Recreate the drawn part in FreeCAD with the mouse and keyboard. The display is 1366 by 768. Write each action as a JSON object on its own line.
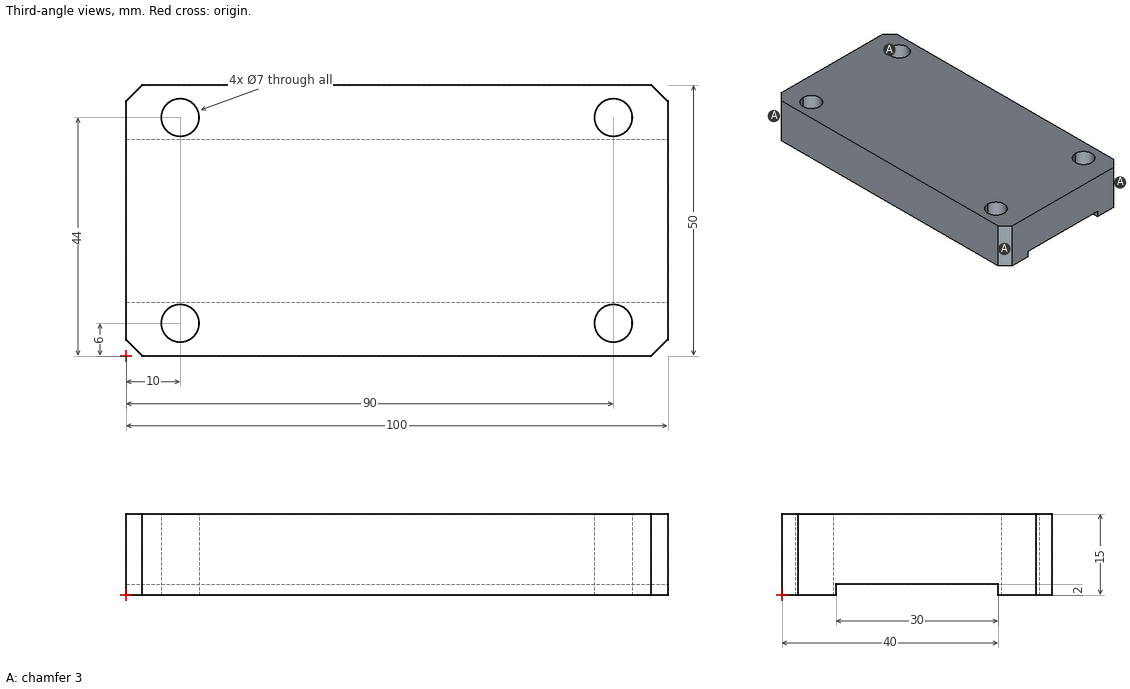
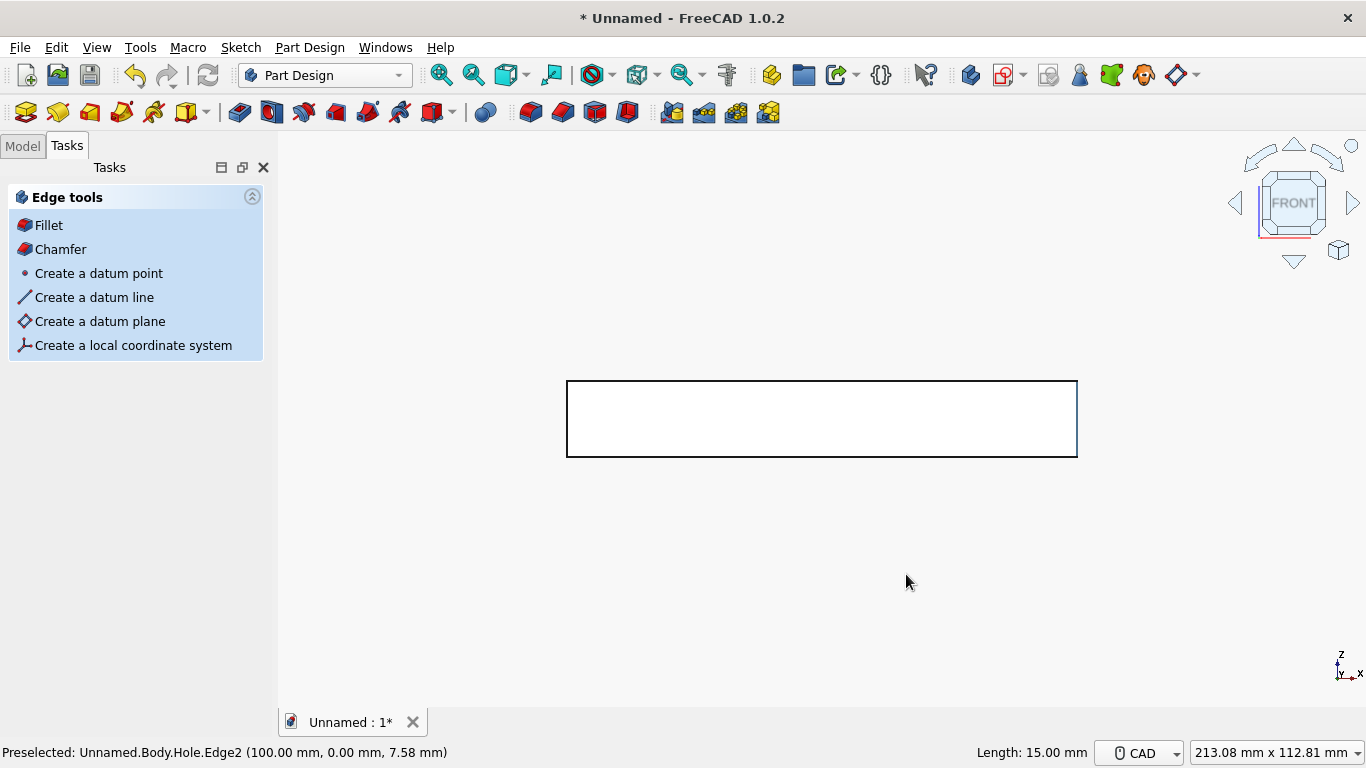
{"action": "left_click", "coordinate": [567, 418], "text": "ctrl"}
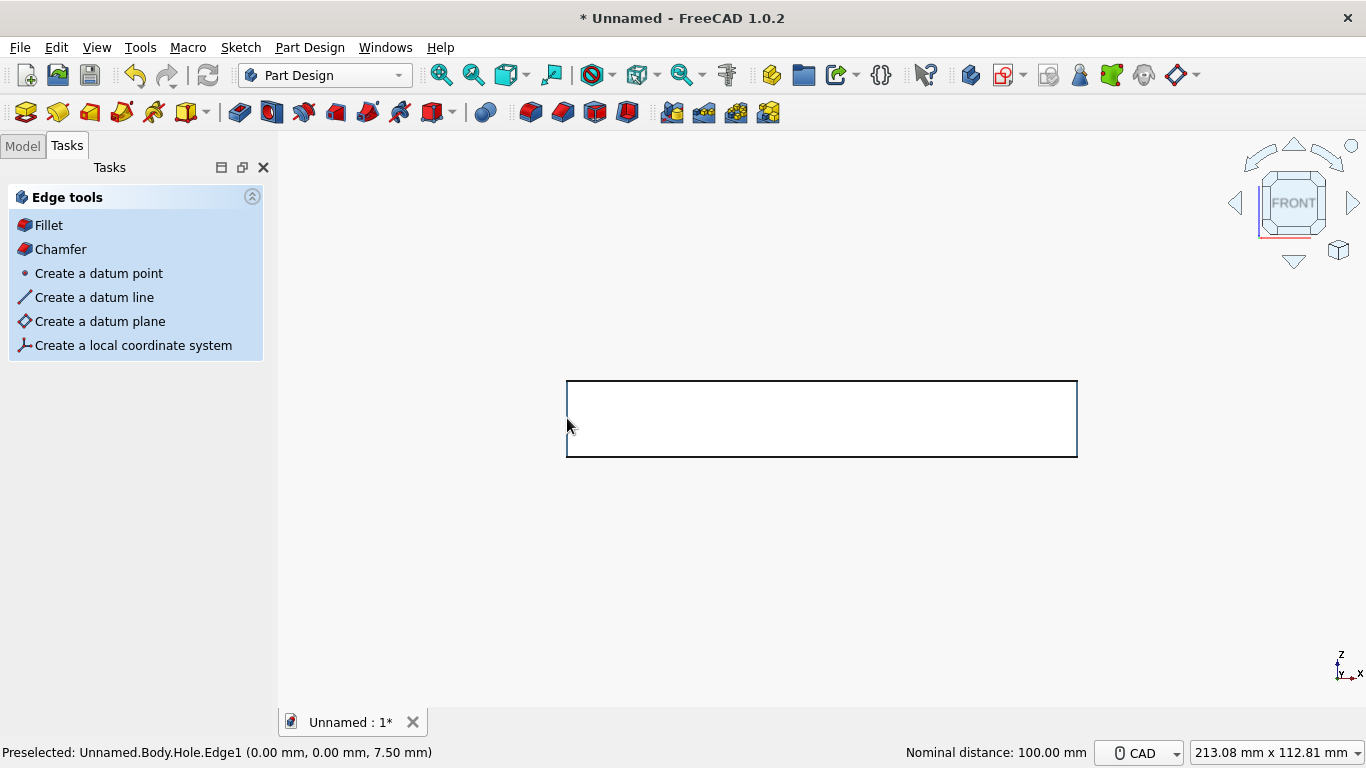
{"action": "key", "text": "3"}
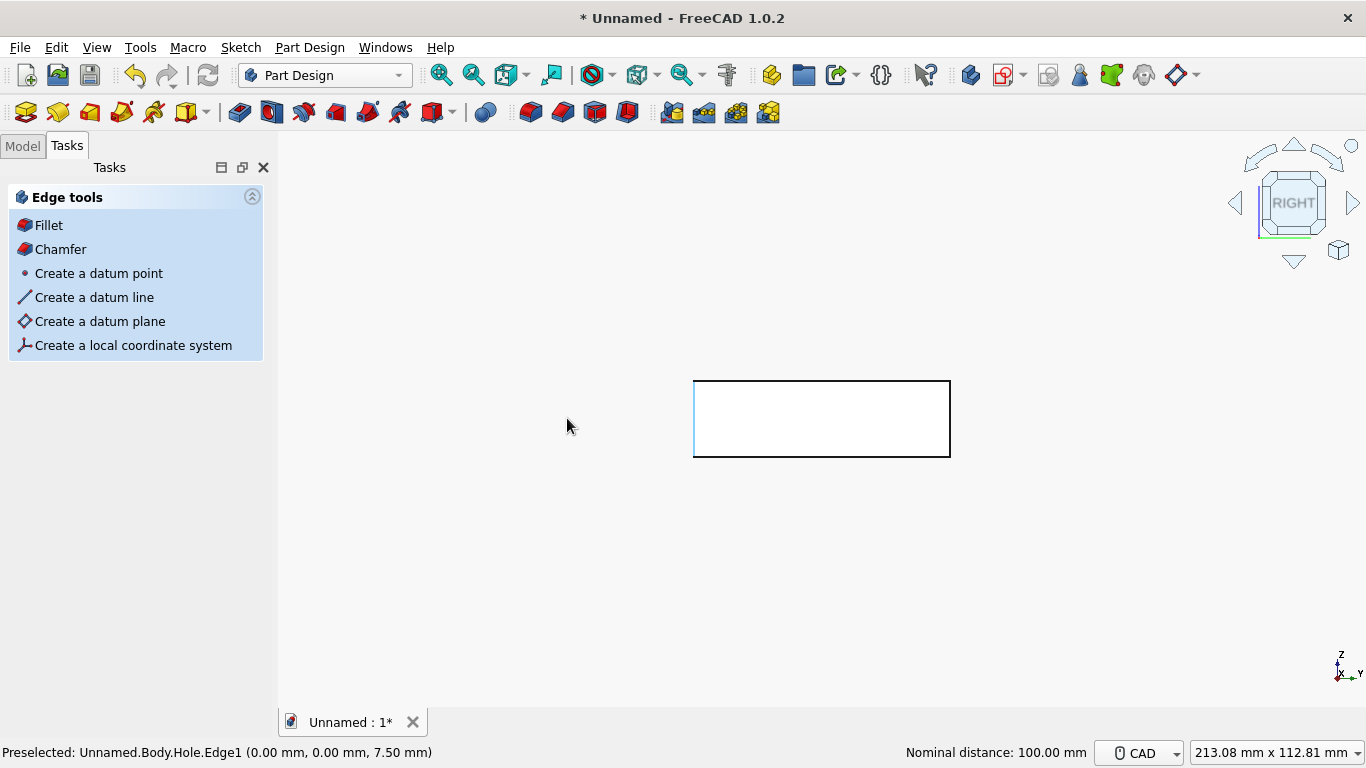
{"action": "key", "text": "v f"}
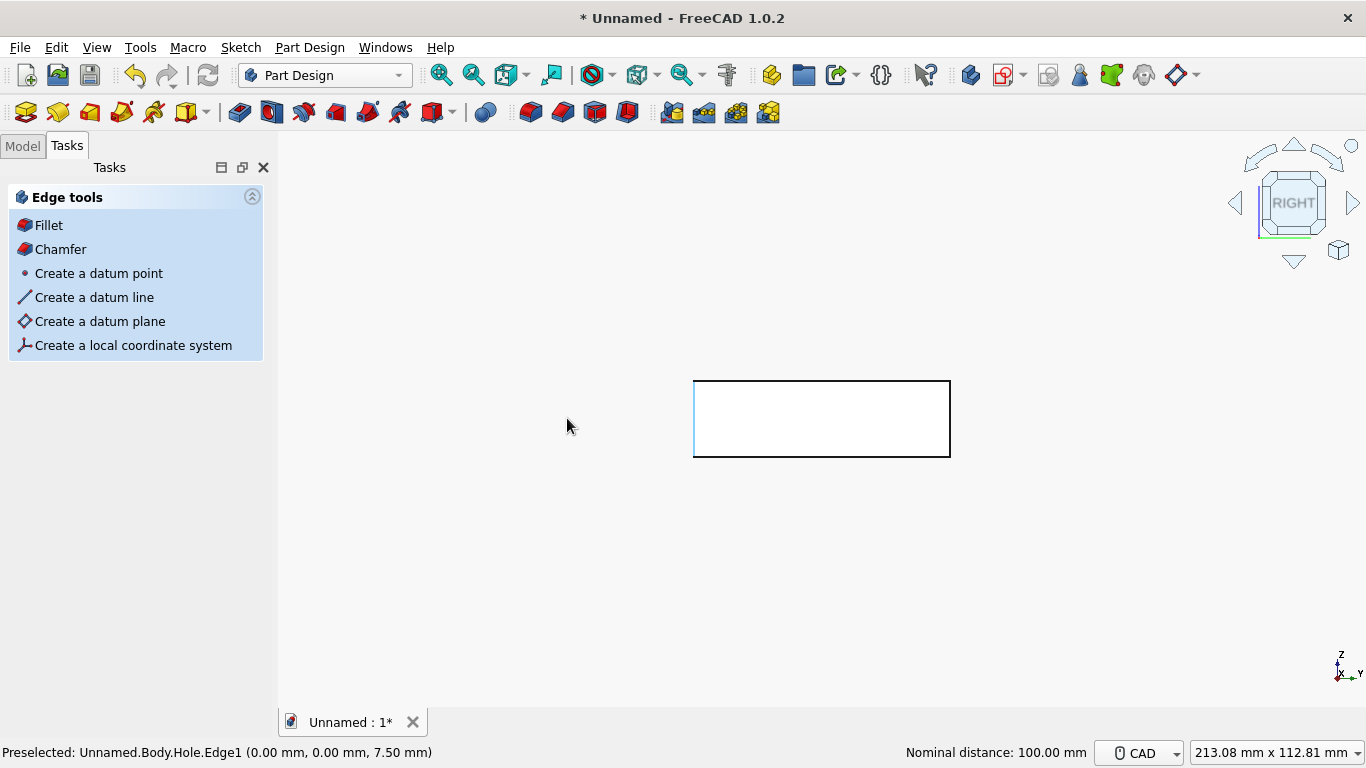
{"action": "left_click", "coordinate": [950, 418], "text": "ctrl"}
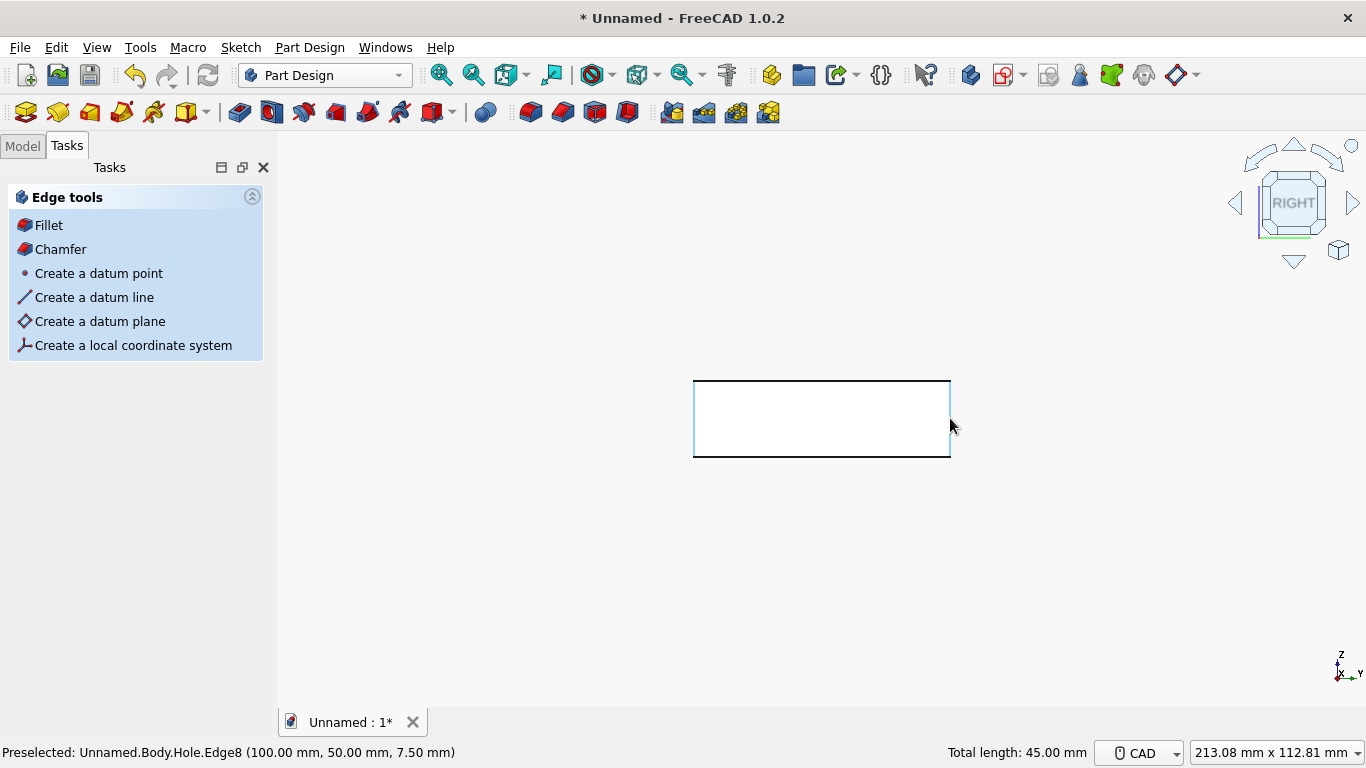
{"action": "key", "text": "5"}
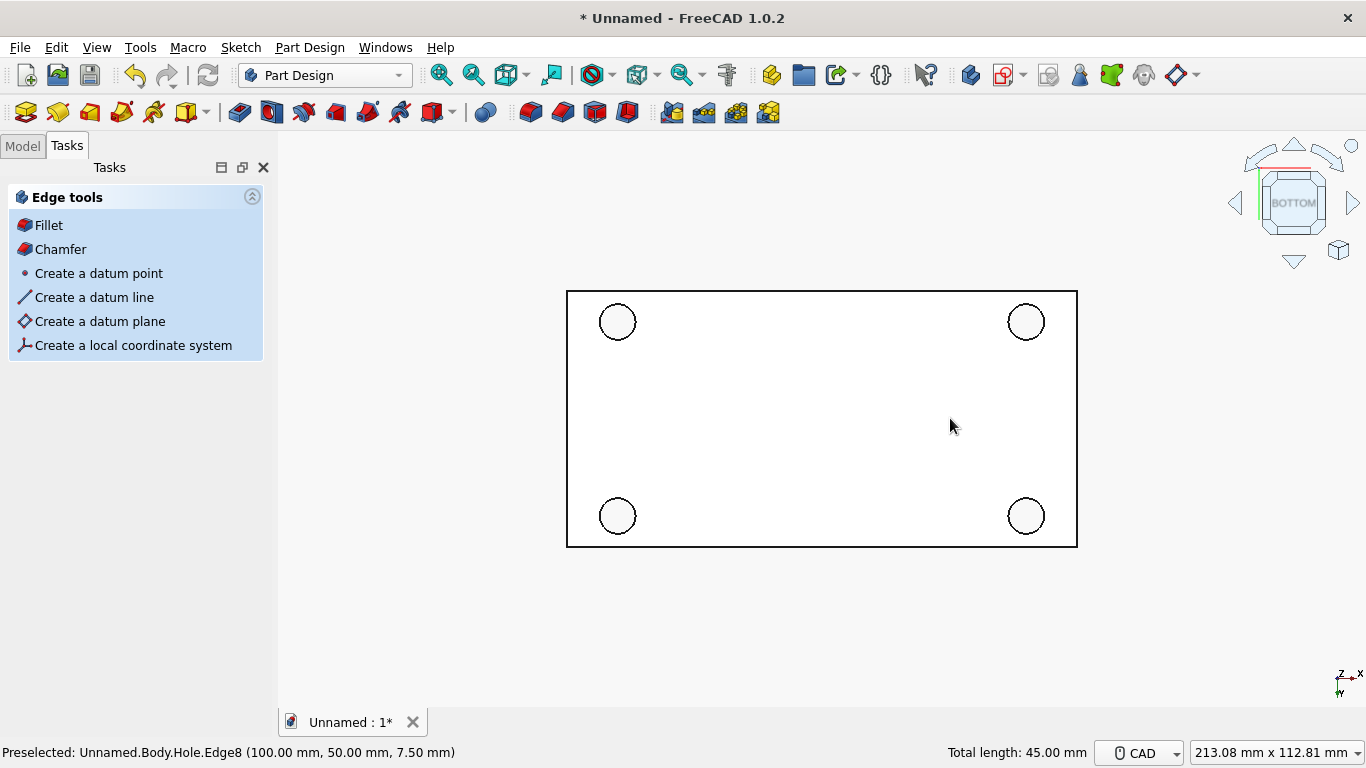
{"action": "key", "text": "4"}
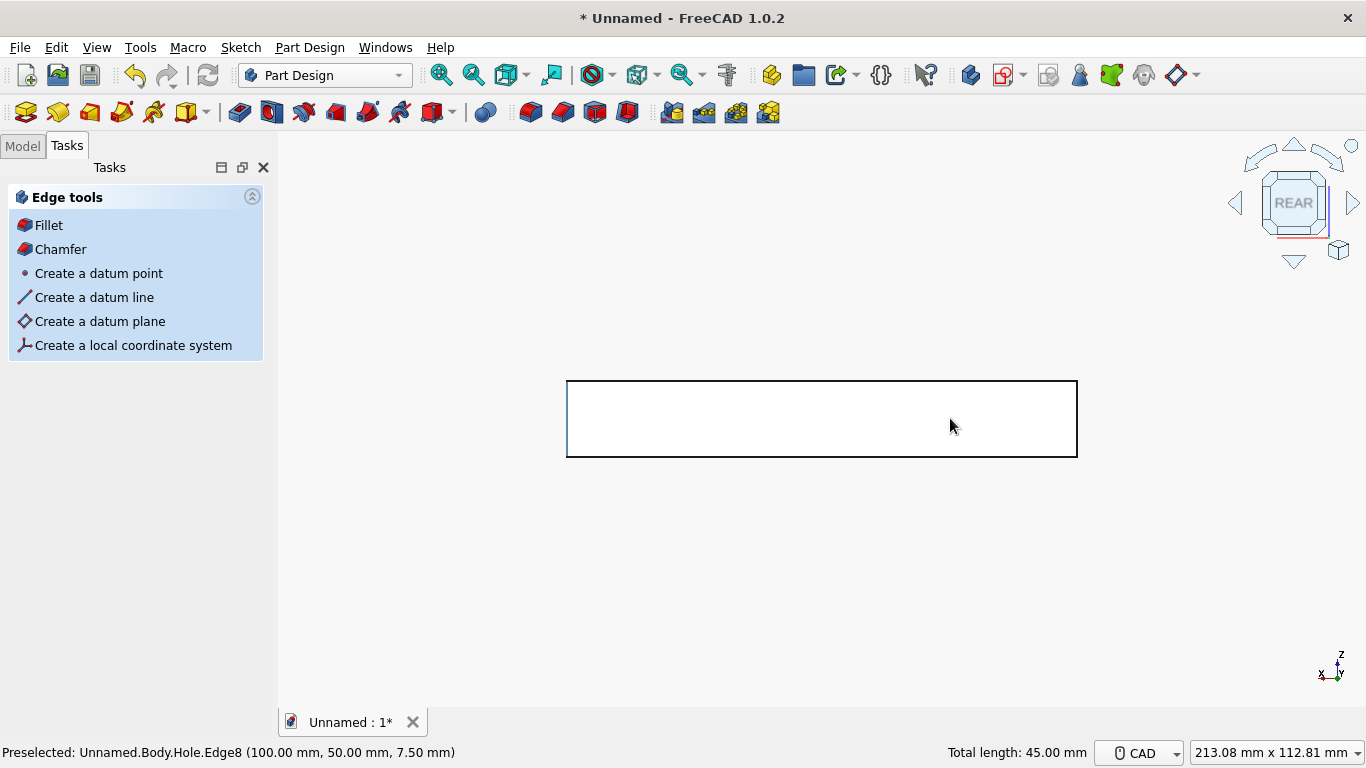
{"action": "left_click", "coordinate": [1077, 418], "text": "ctrl"}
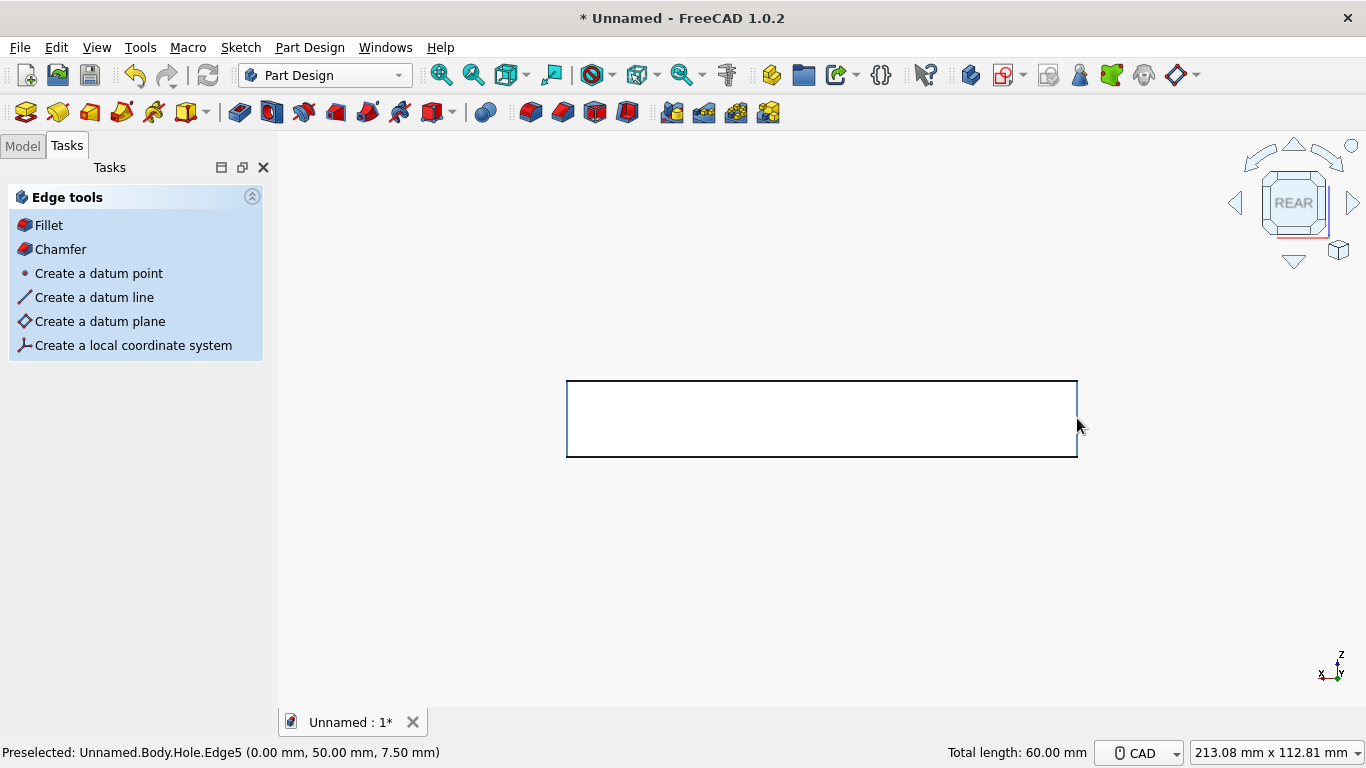
{"action": "left_click", "coordinate": [564, 112]}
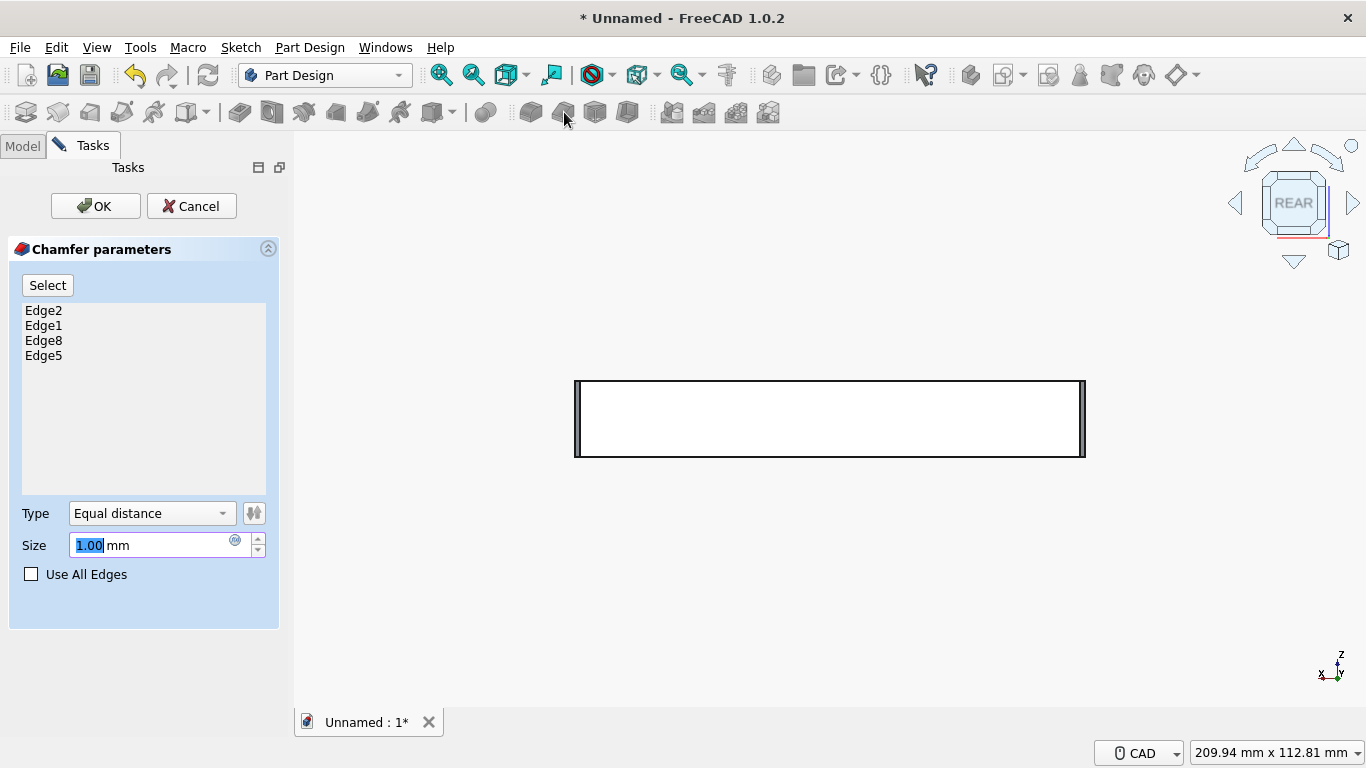
{"action": "type", "text": "3"}
{"action": "key", "text": "Tab"}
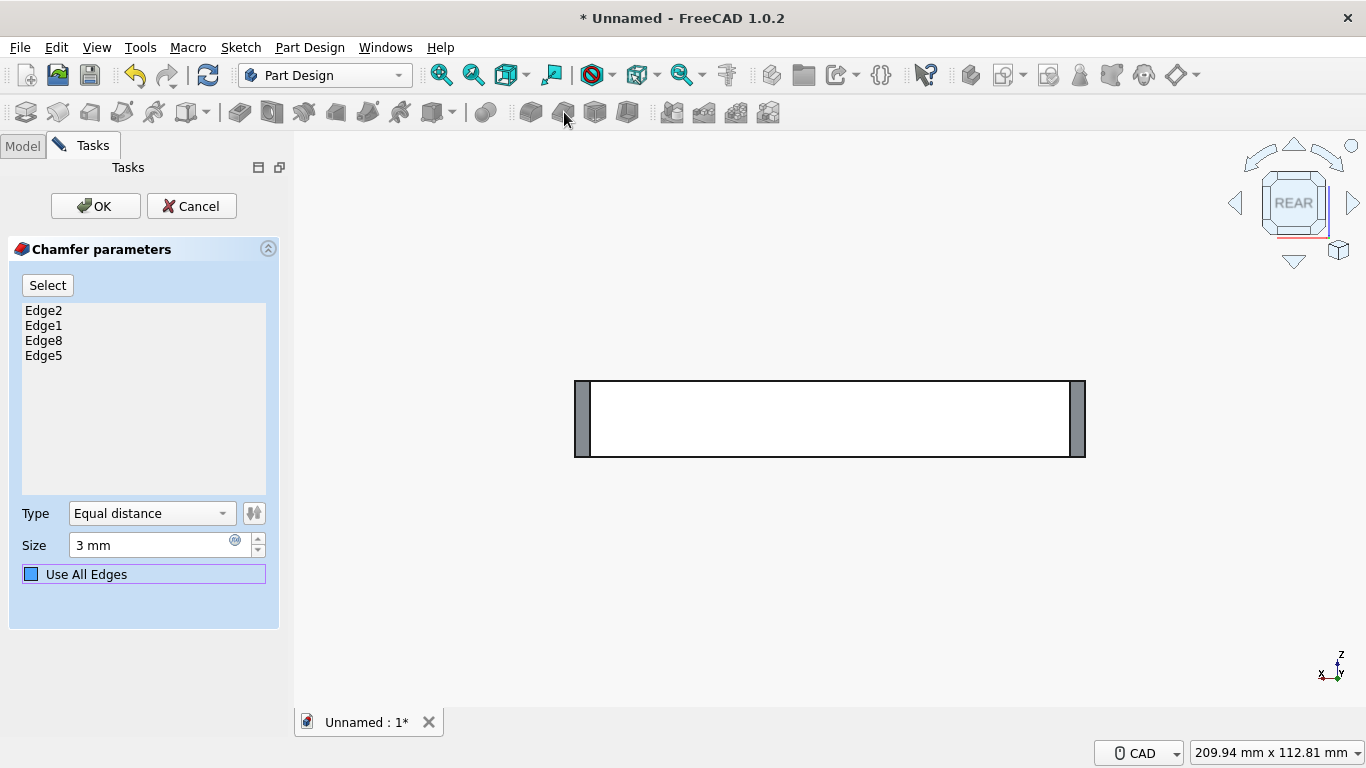
{"action": "left_click", "coordinate": [96, 206]}